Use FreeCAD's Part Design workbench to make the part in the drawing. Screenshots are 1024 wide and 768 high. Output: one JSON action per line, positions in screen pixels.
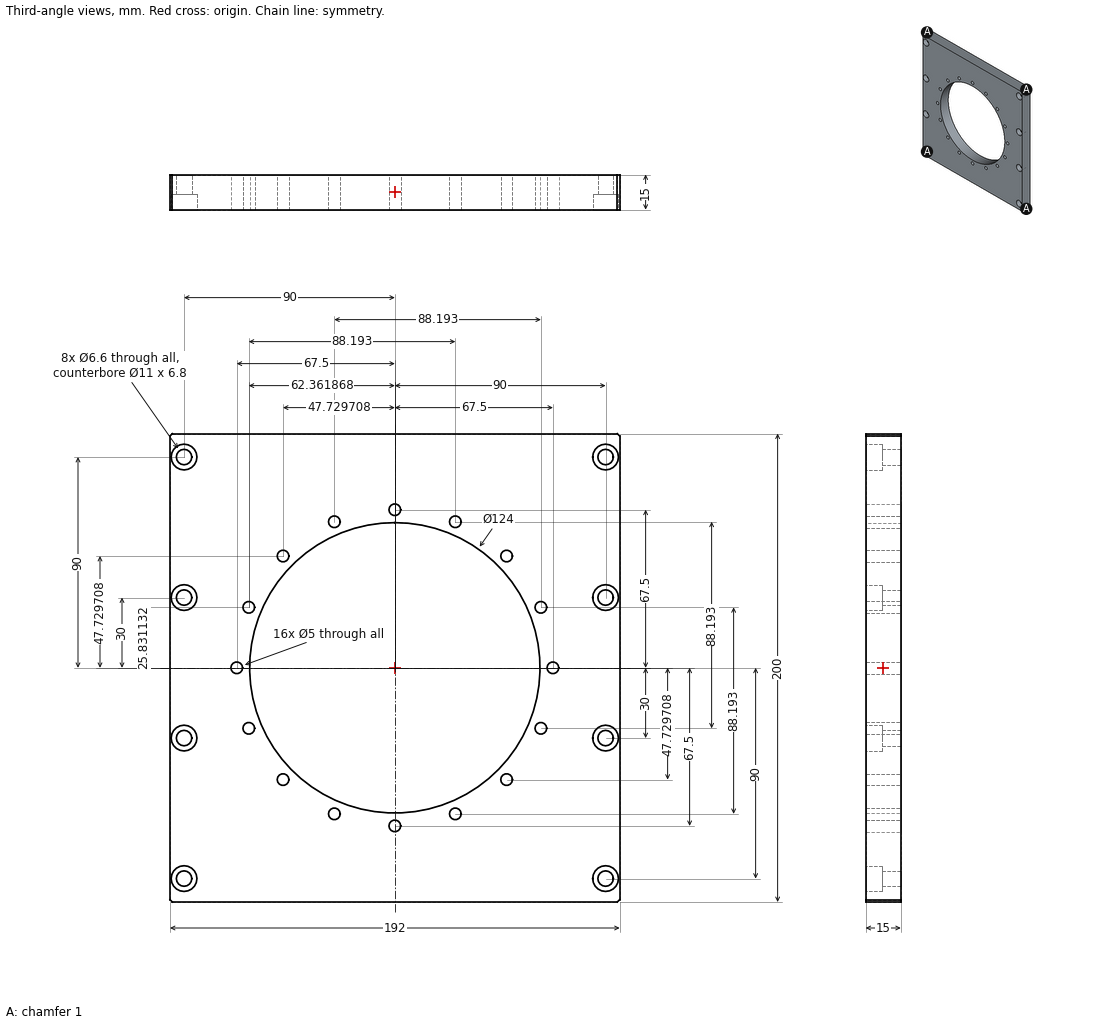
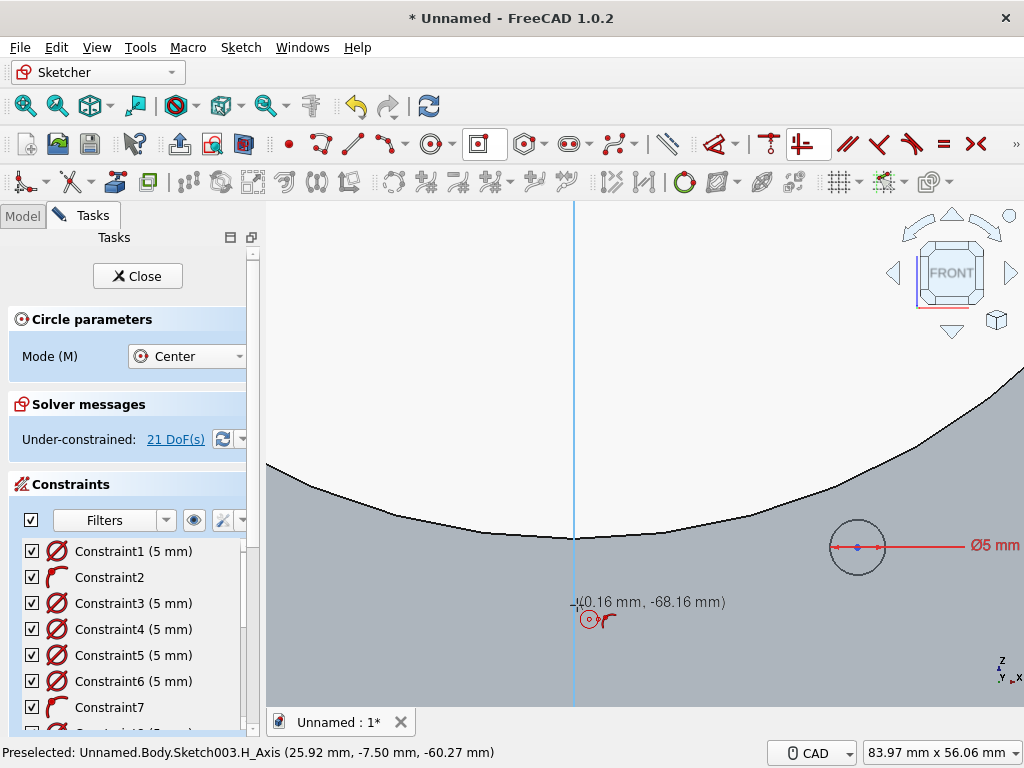
{"action": "scroll", "coordinate": [577, 605], "scroll_direction": "down", "scroll_amount": 8}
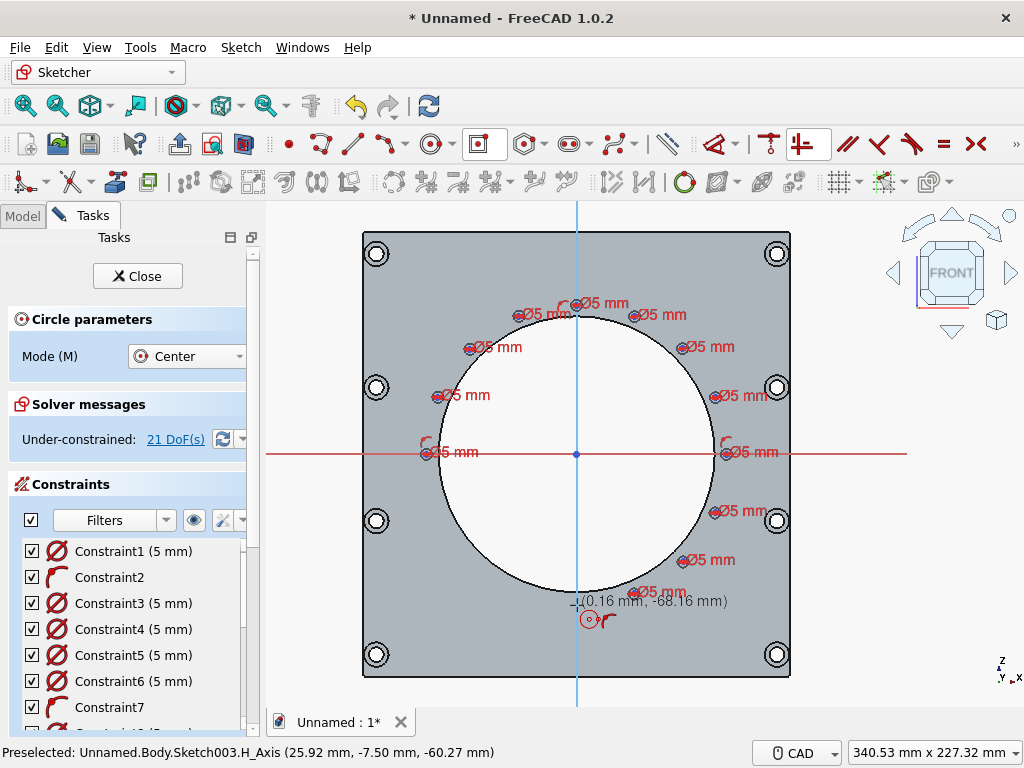
{"action": "left_click", "coordinate": [577, 605]}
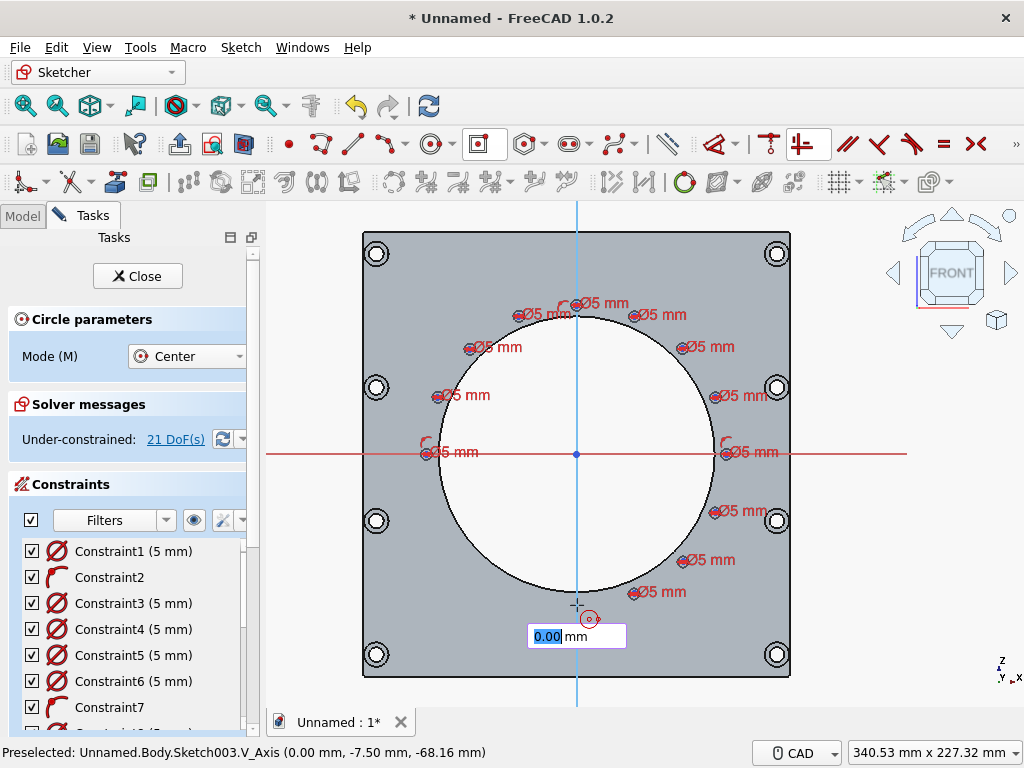
{"action": "scroll", "coordinate": [582, 603], "scroll_direction": "up", "scroll_amount": 6}
{"action": "mouse_move", "coordinate": [581, 600]}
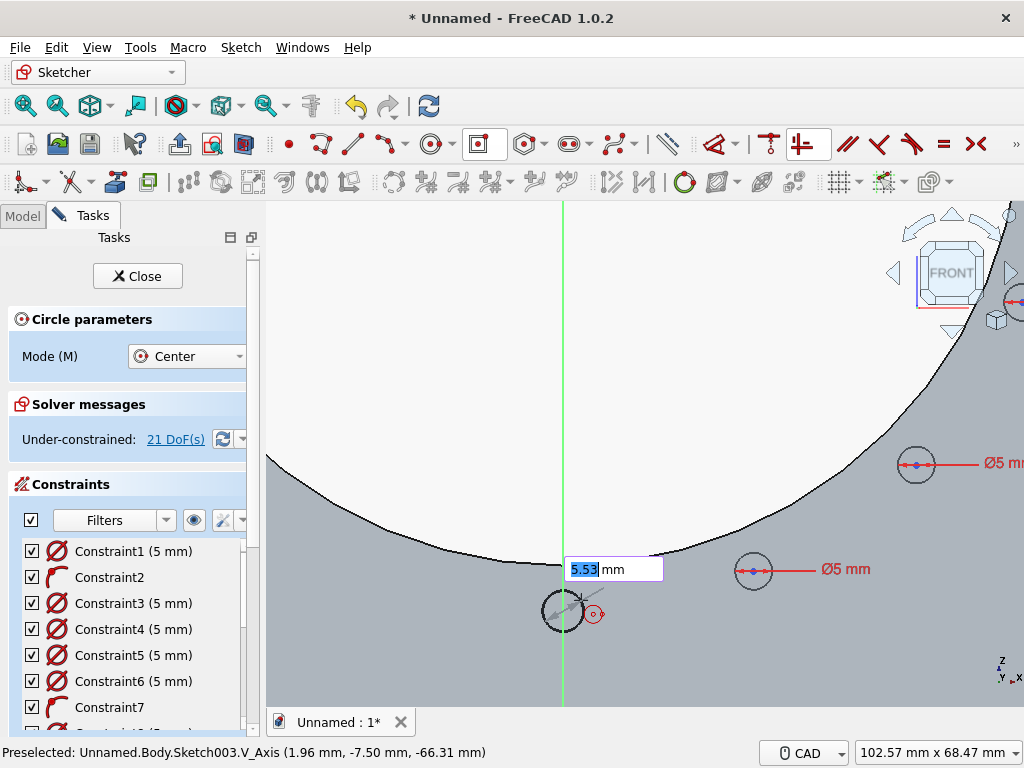
{"action": "type", "text": "5"}
{"action": "key", "text": "Return"}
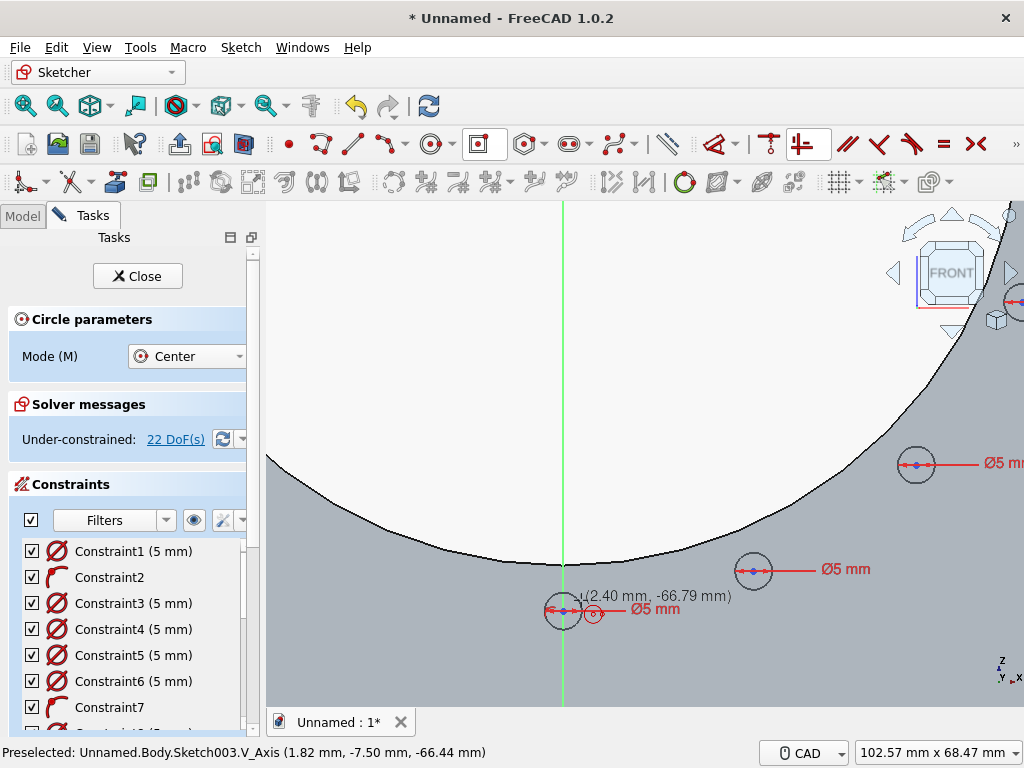
{"action": "scroll", "coordinate": [372, 568], "scroll_direction": "up", "scroll_amount": 2}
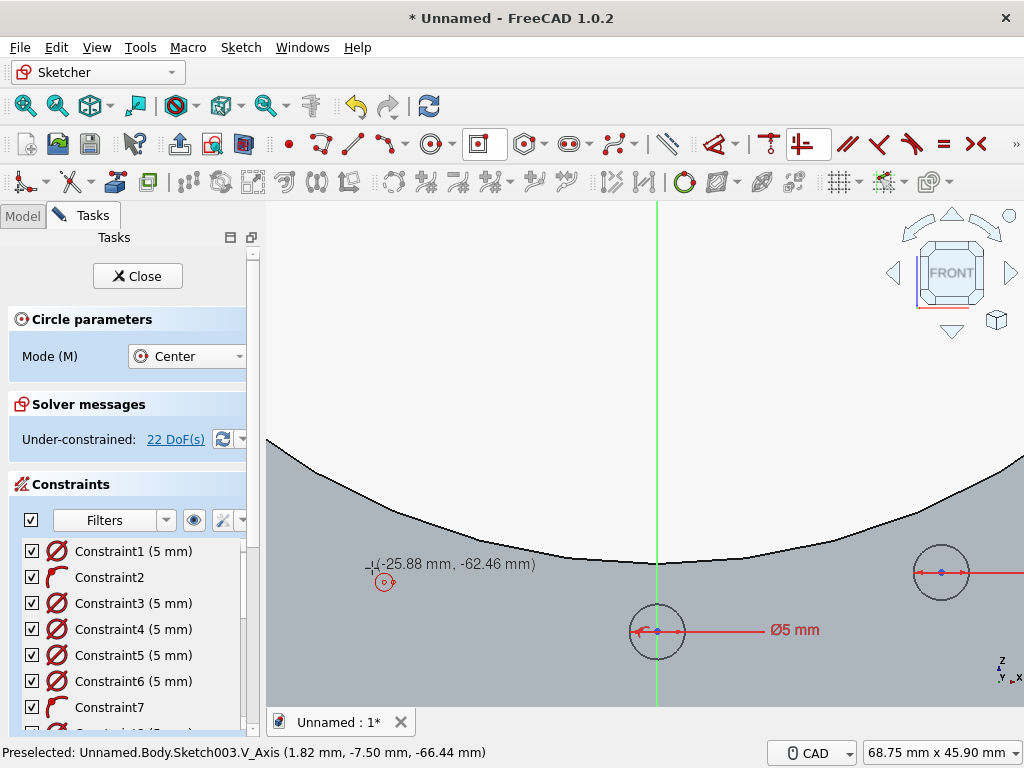
{"action": "scroll", "coordinate": [556, 599], "scroll_direction": "down", "scroll_amount": 8}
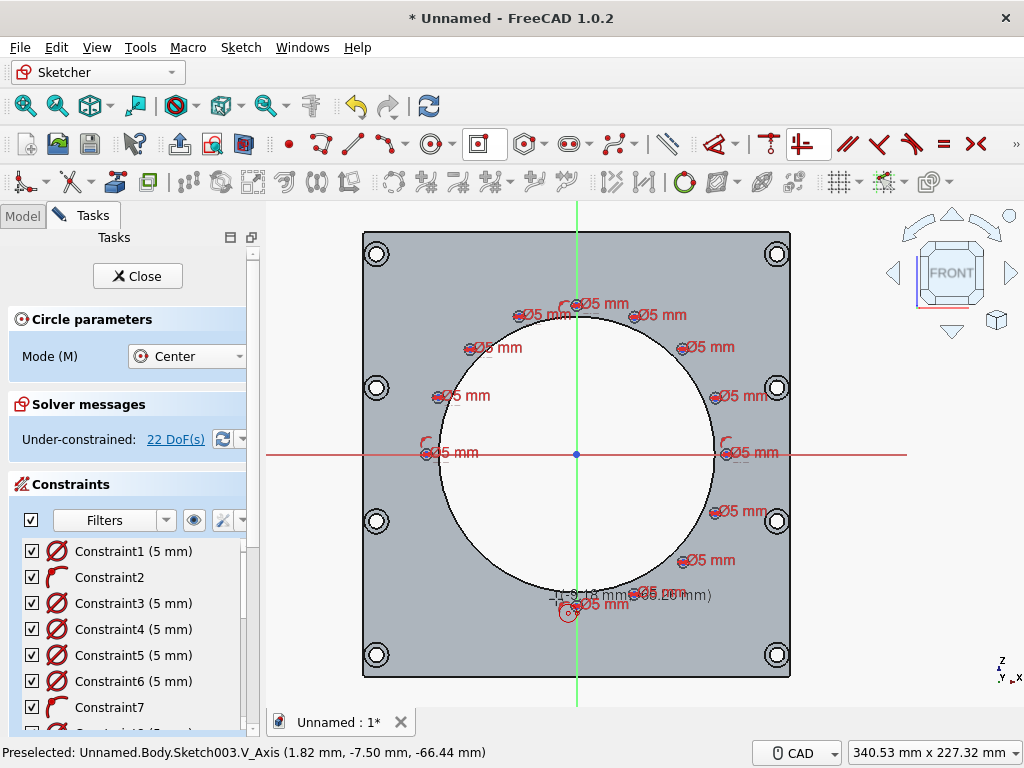
{"action": "left_click", "coordinate": [519, 593]}
{"action": "mouse_move", "coordinate": [523, 589]}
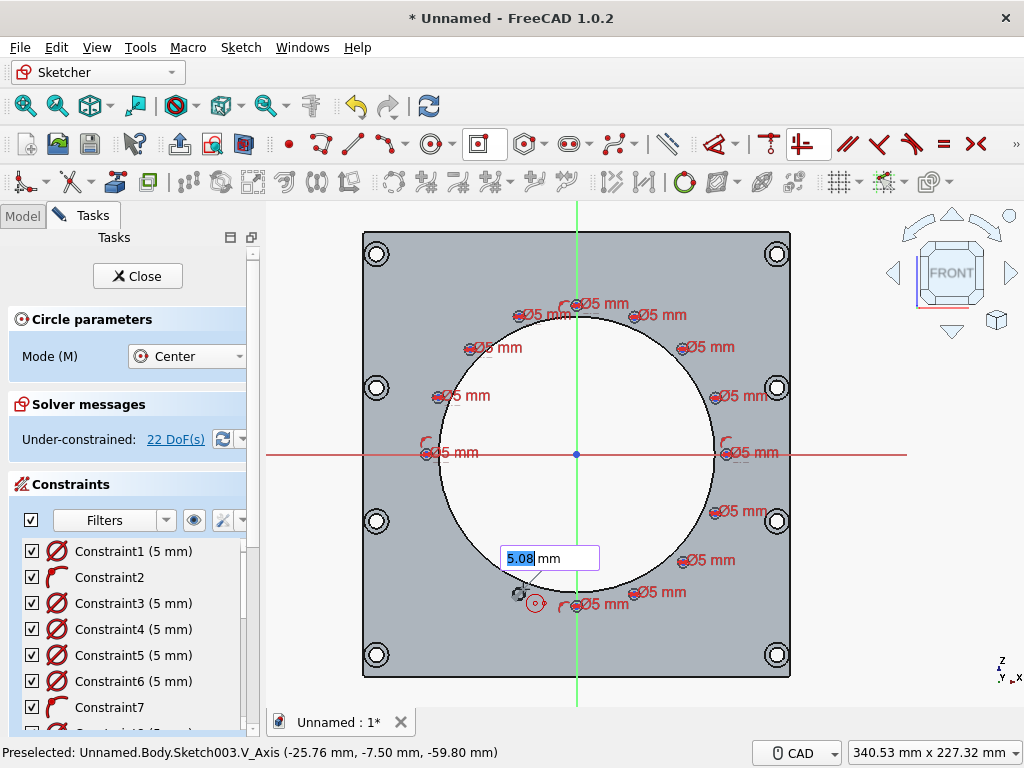
{"action": "type", "text": "5"}
{"action": "key", "text": "Return"}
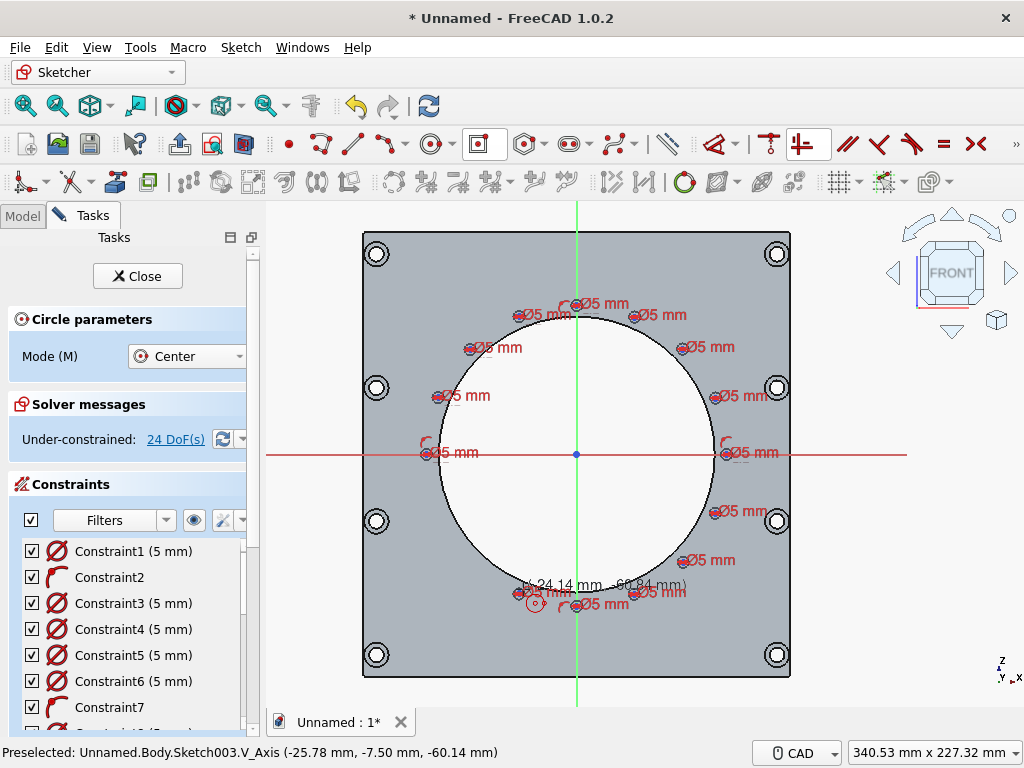
{"action": "scroll", "coordinate": [471, 561], "scroll_direction": "up", "scroll_amount": 8}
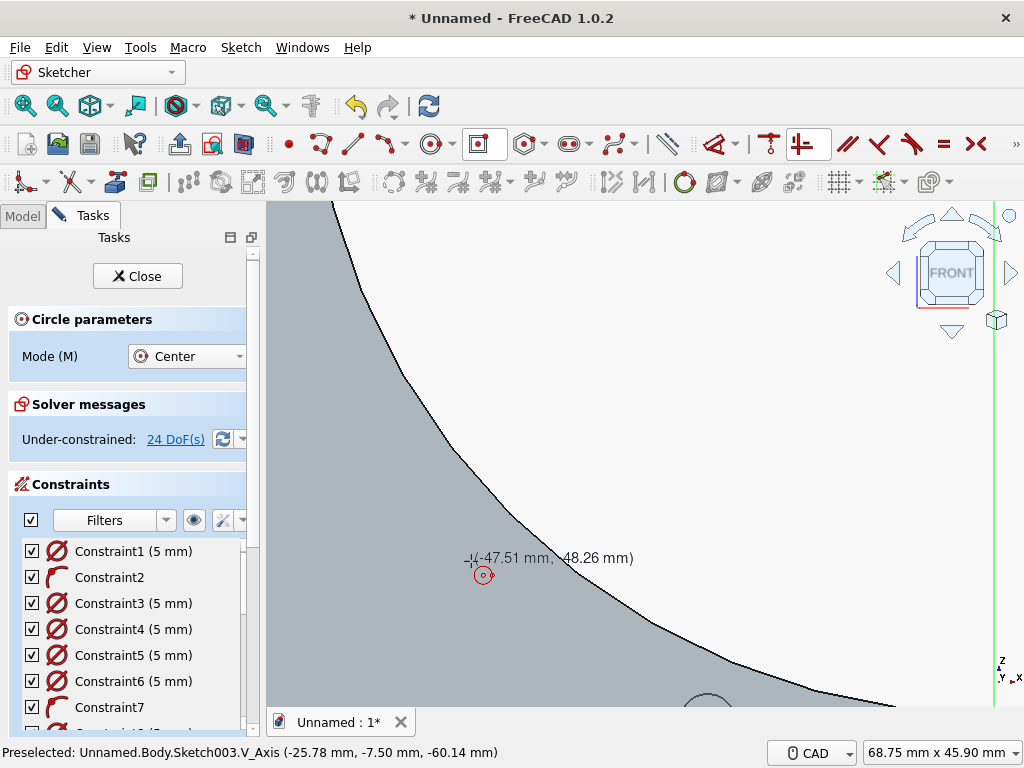
{"action": "scroll", "coordinate": [471, 561], "scroll_direction": "down", "scroll_amount": 8}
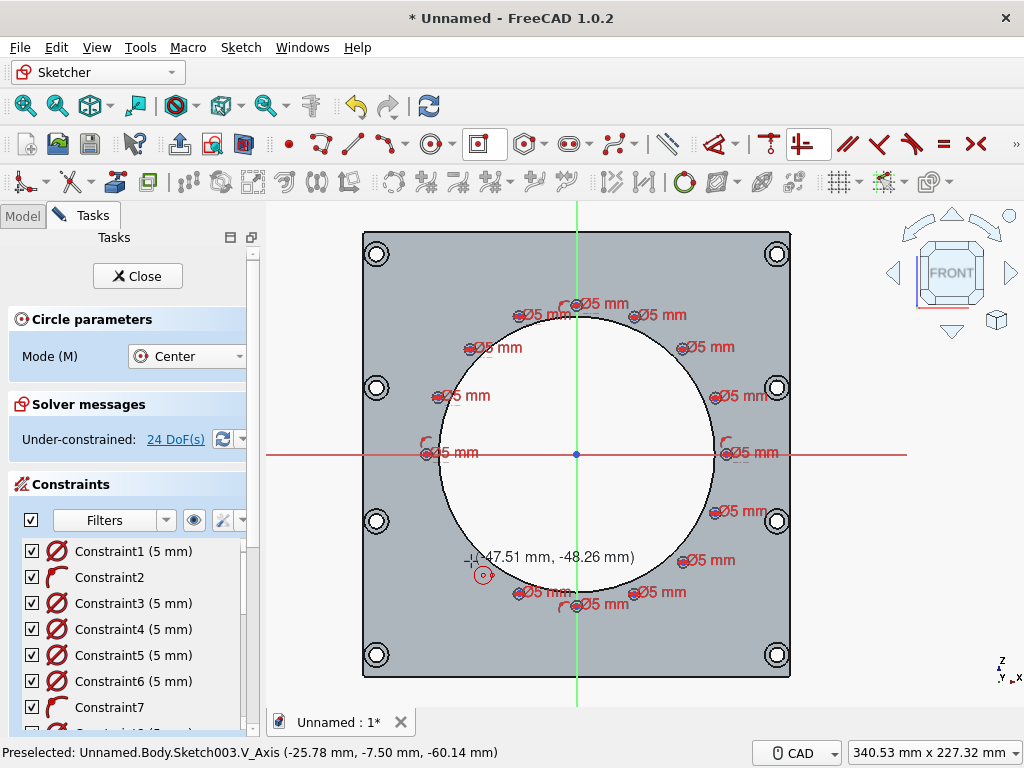
{"action": "left_click", "coordinate": [471, 561]}
{"action": "mouse_move", "coordinate": [474, 557]}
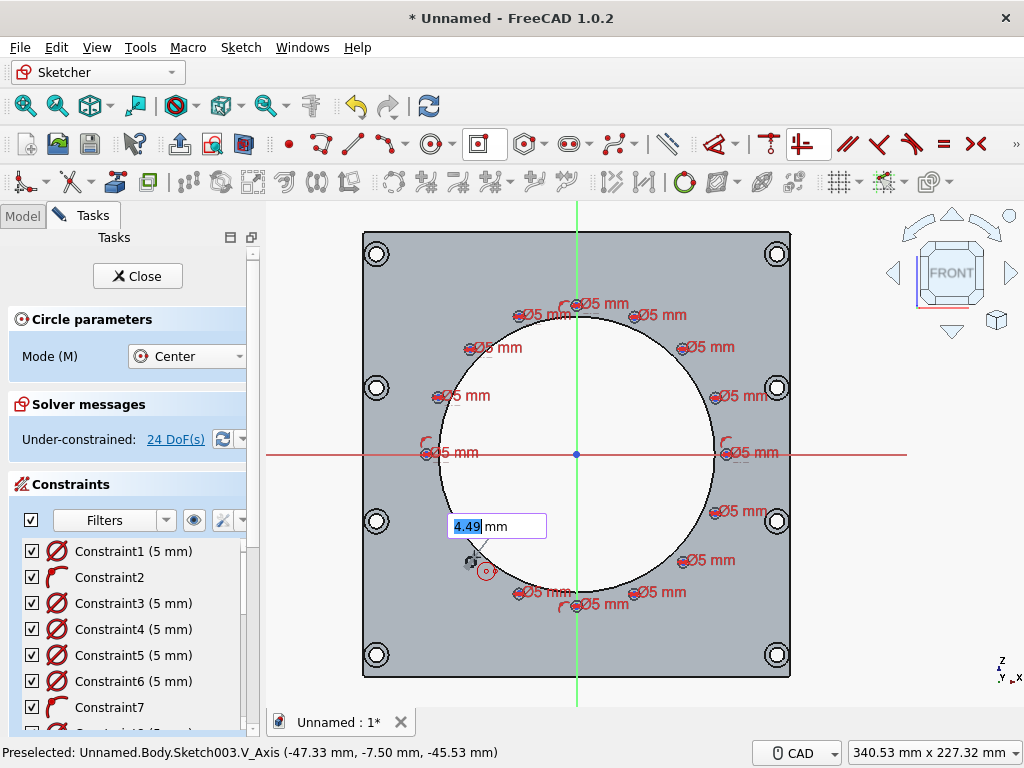
{"action": "type", "text": "5"}
{"action": "key", "text": "Return"}